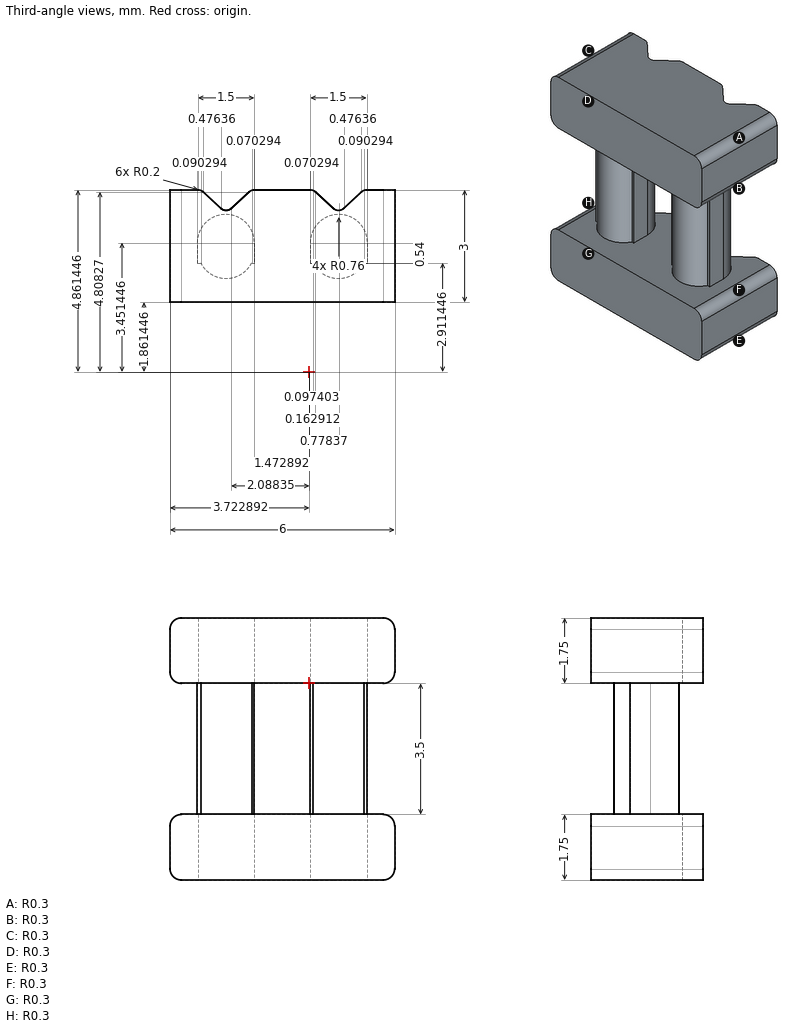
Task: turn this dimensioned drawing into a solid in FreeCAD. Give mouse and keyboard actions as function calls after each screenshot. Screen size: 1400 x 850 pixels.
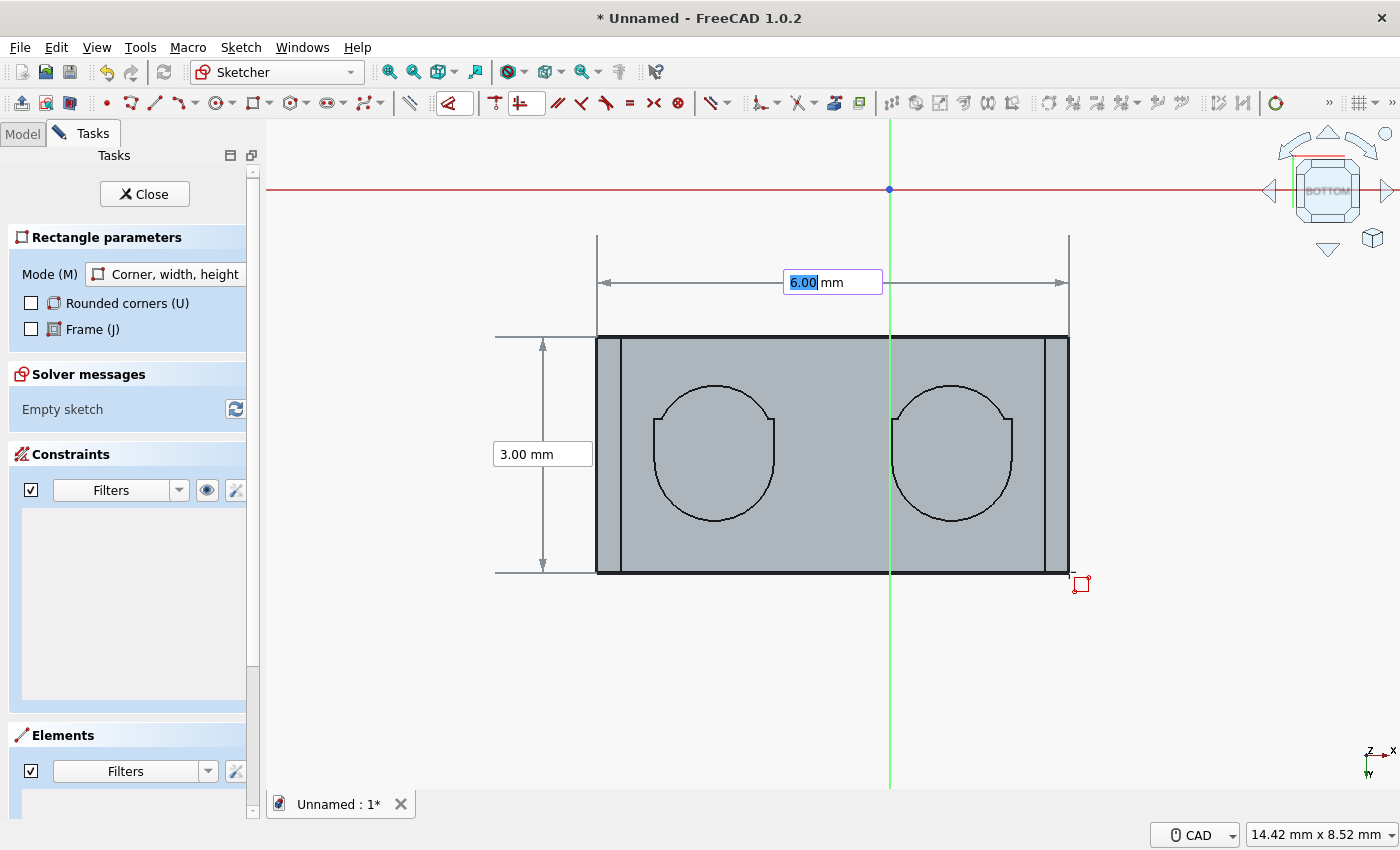
text(6)
key(Tab)
text(3)
key(Return)
key(Escape)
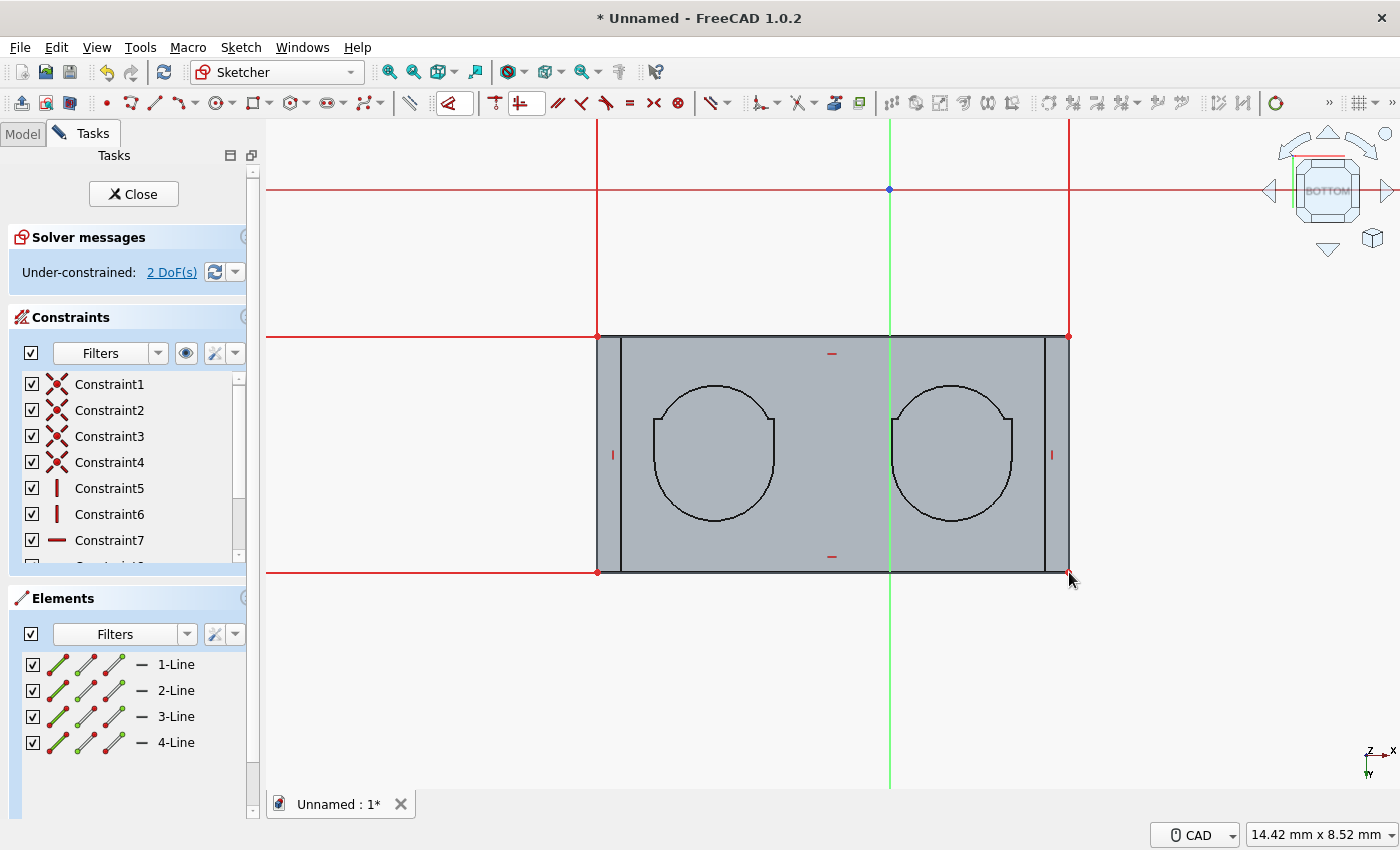
click(597, 337)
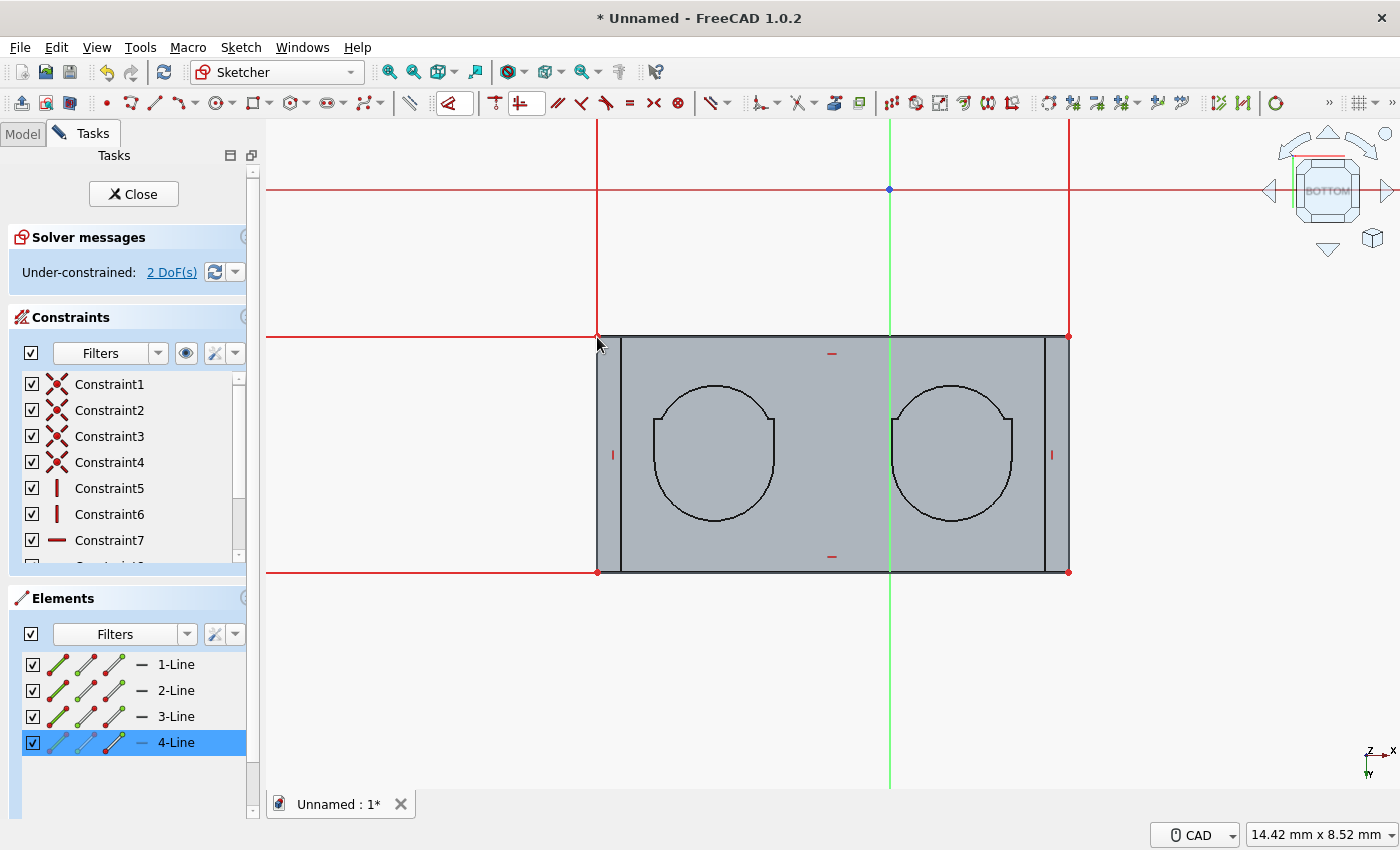
click(468, 104)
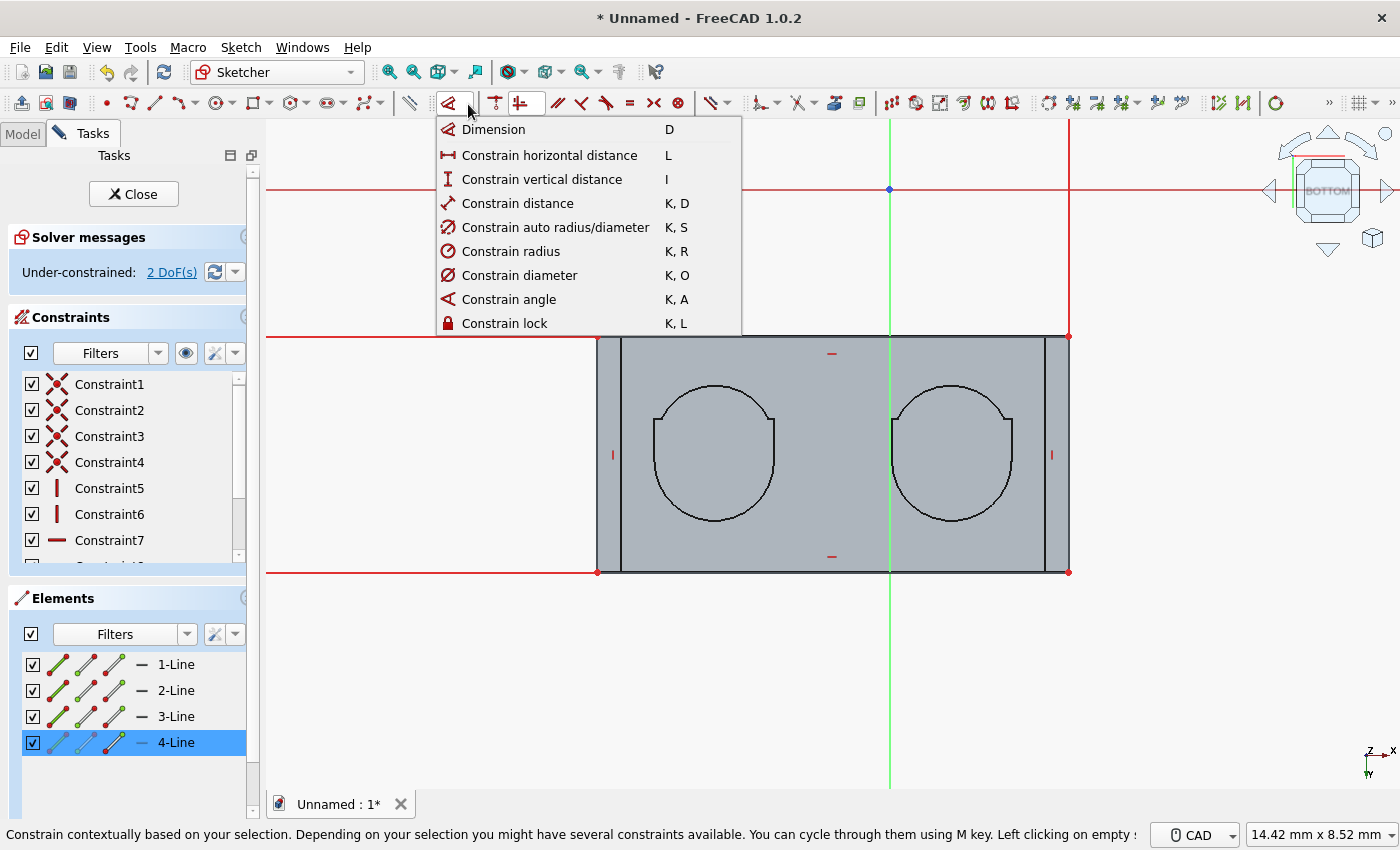
click(589, 155)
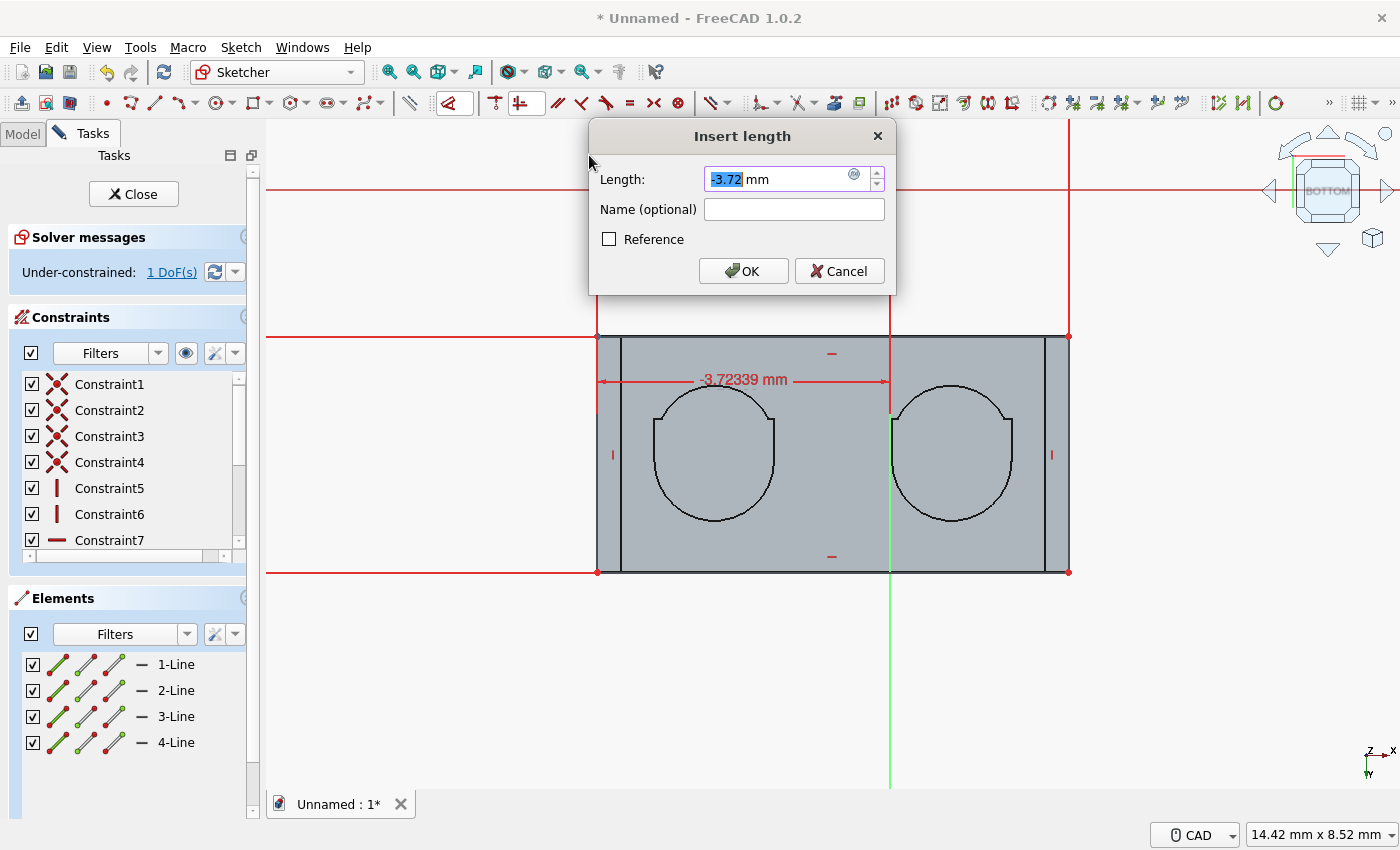
text(-3.722892)
key(Return)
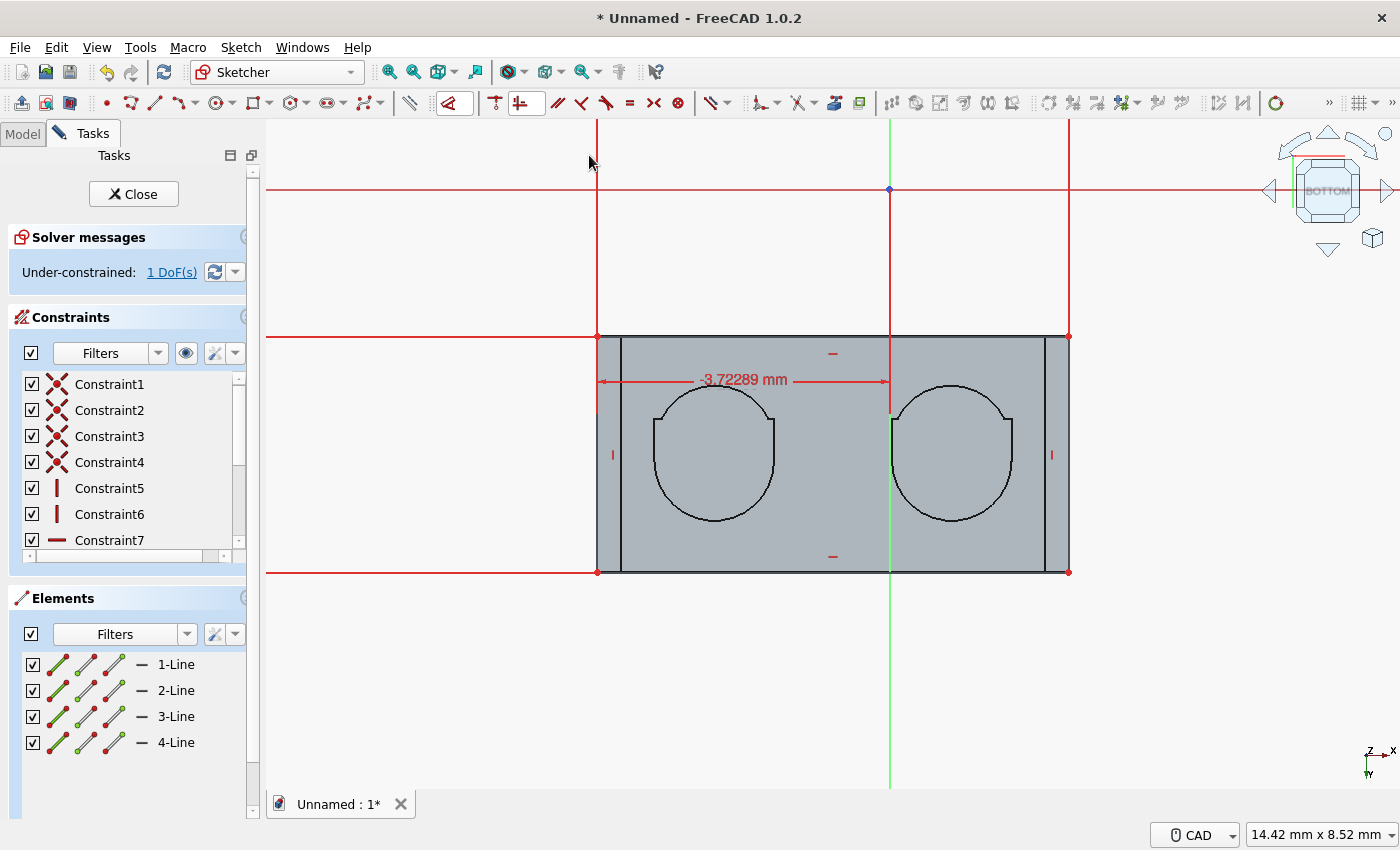
click(597, 337)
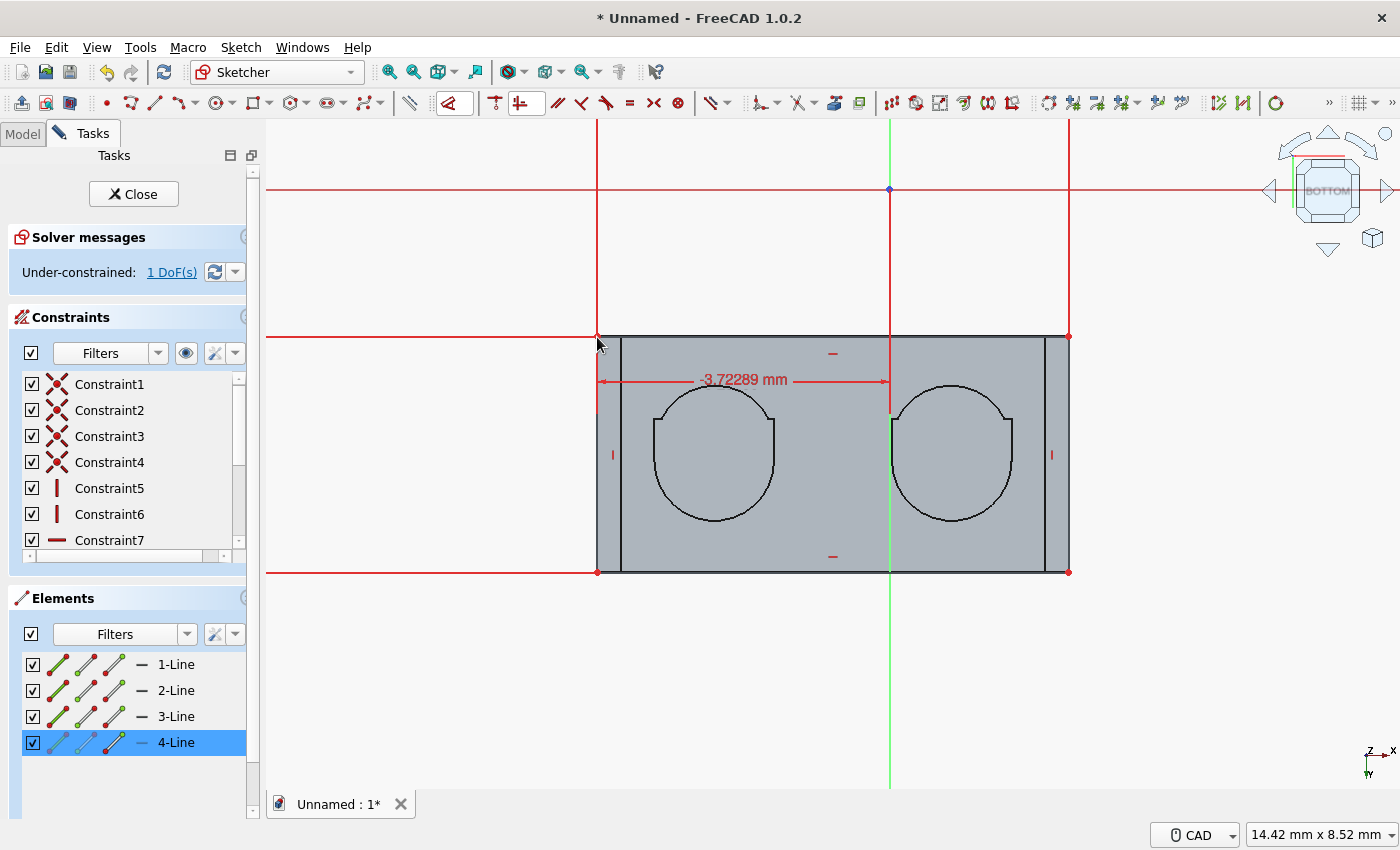
key(i)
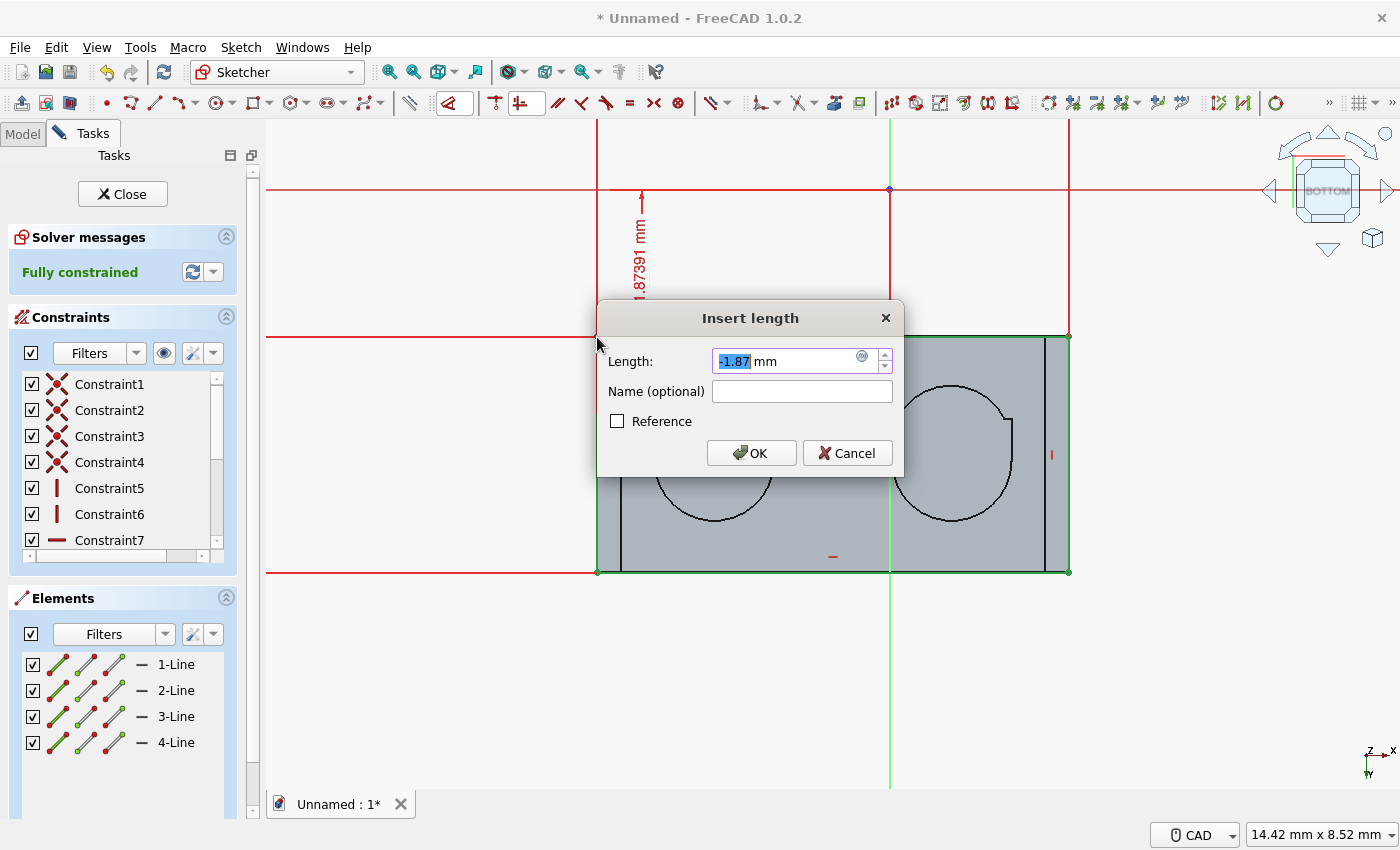
text(-1.861446)
key(Return)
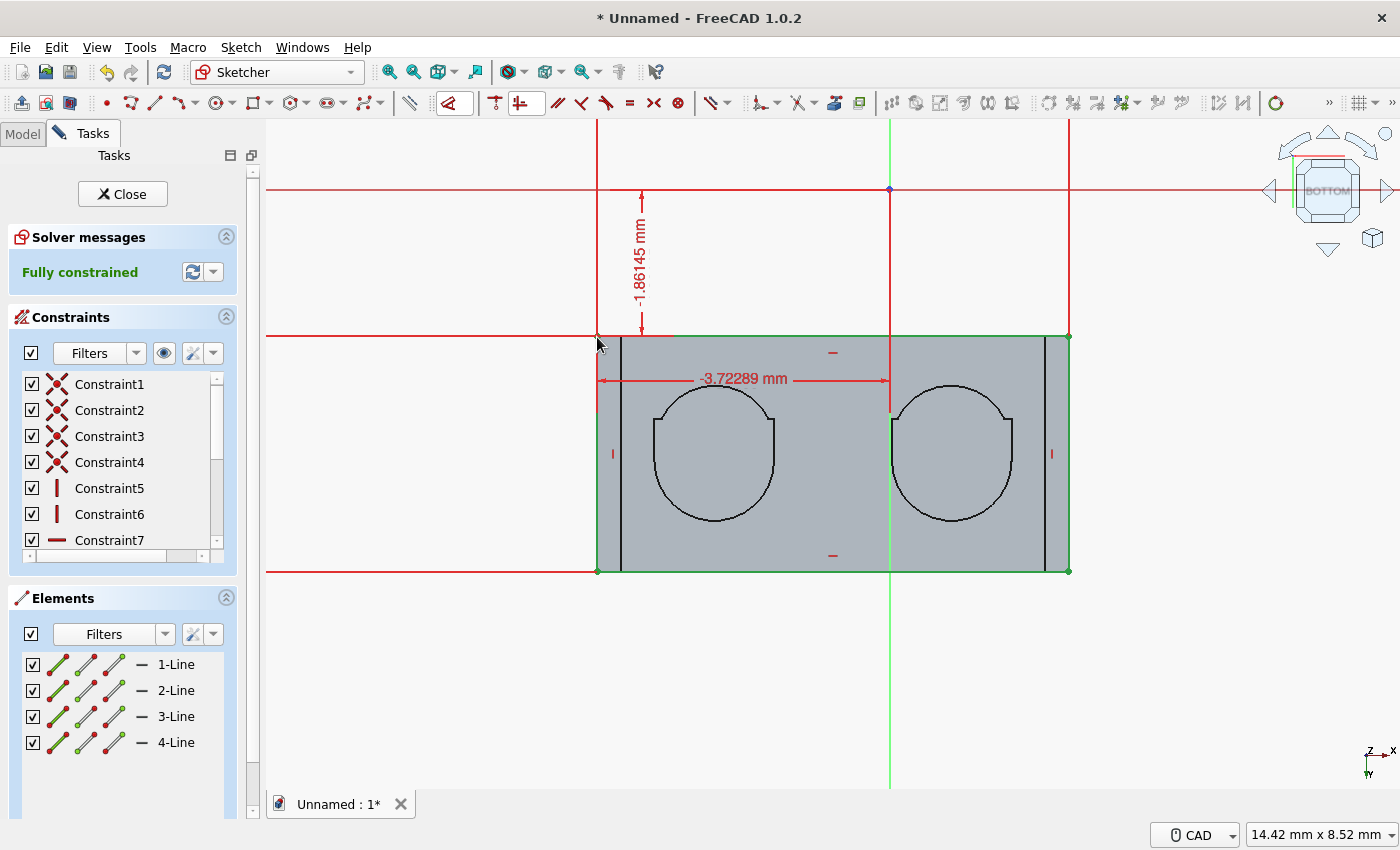
click(123, 194)